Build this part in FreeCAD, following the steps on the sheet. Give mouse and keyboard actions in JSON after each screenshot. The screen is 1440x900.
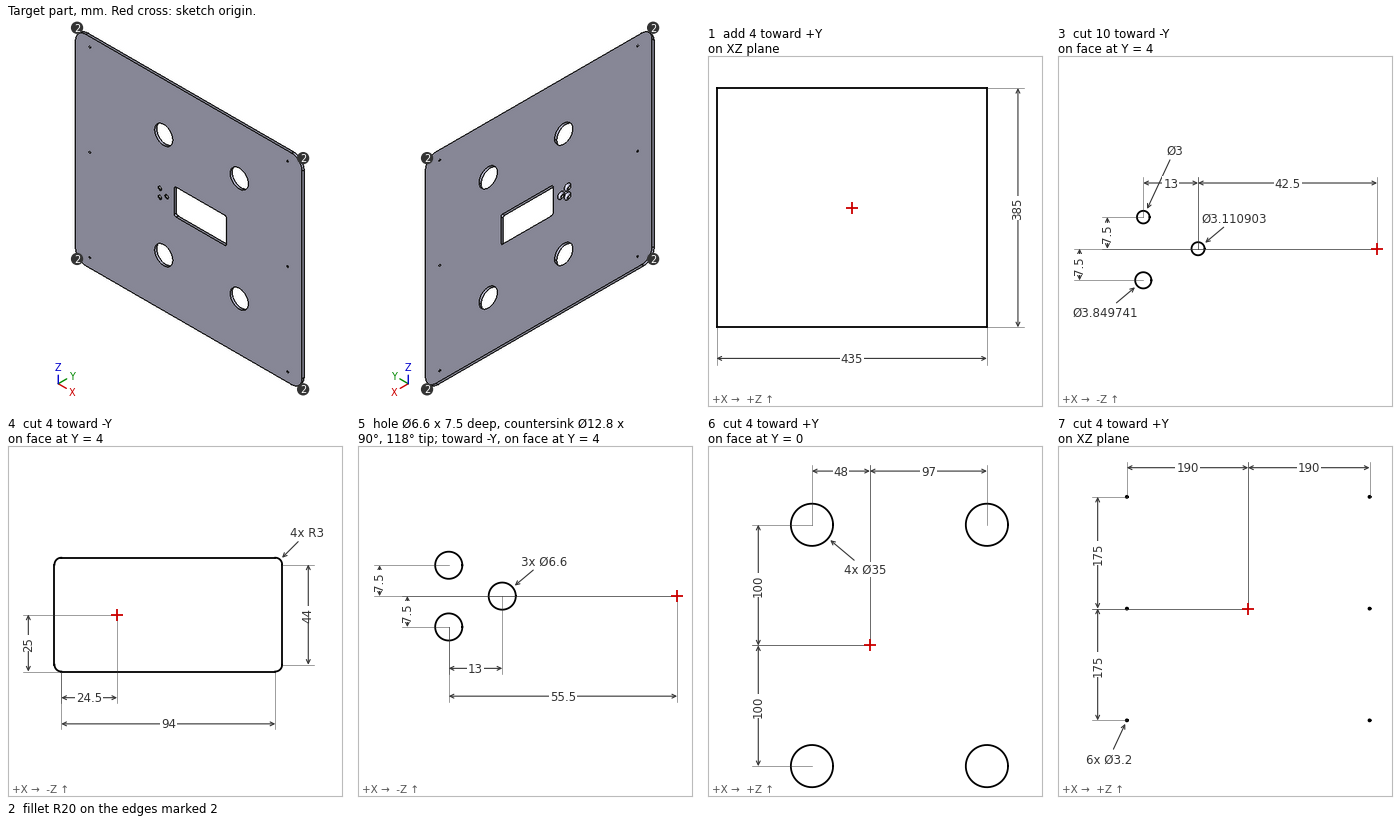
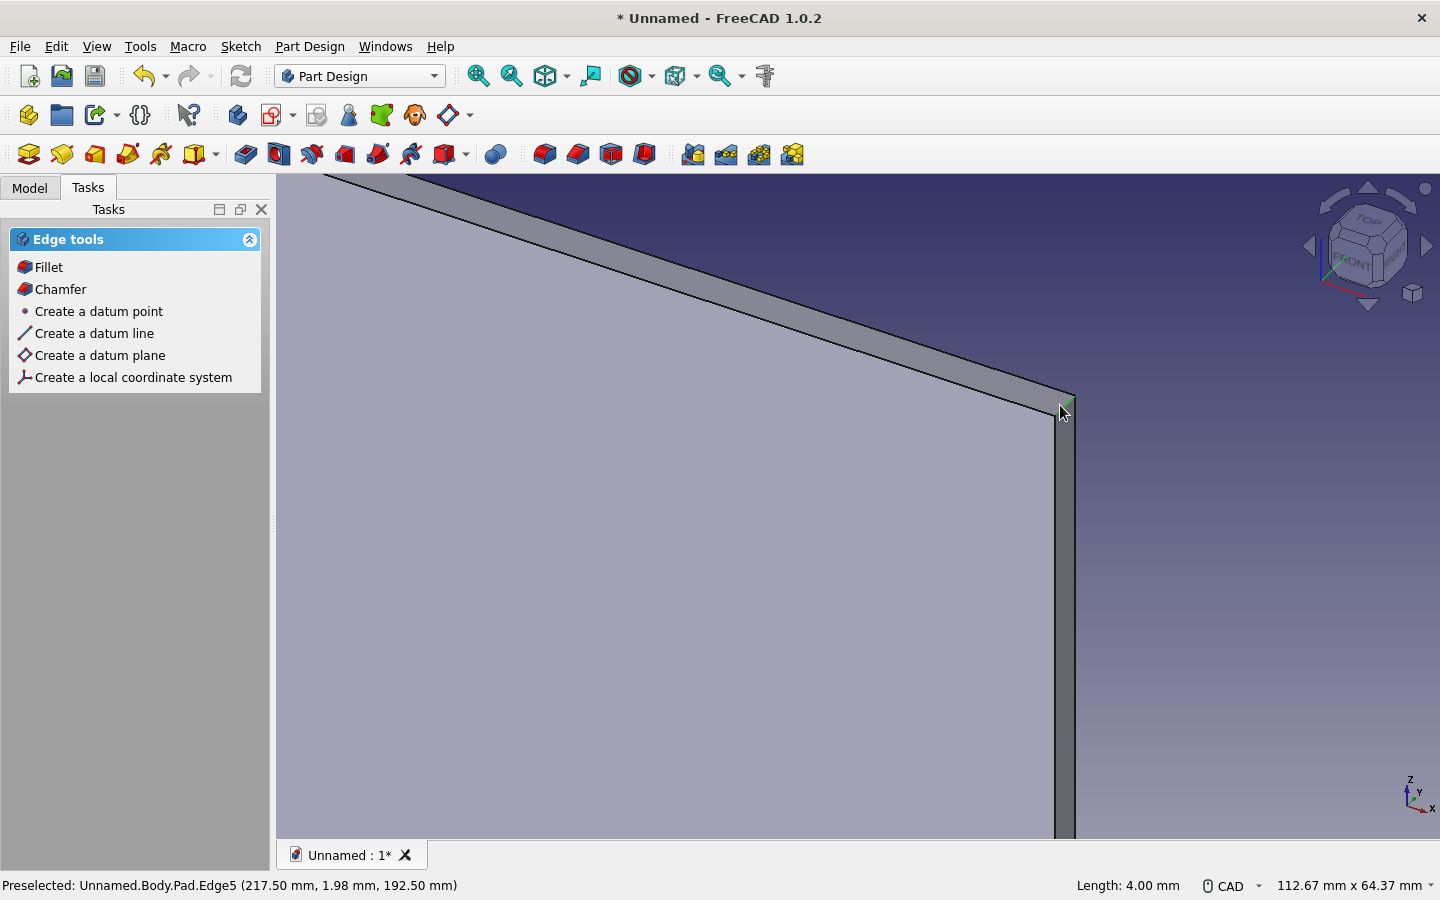
{"action": "left_click", "coordinate": [479, 76]}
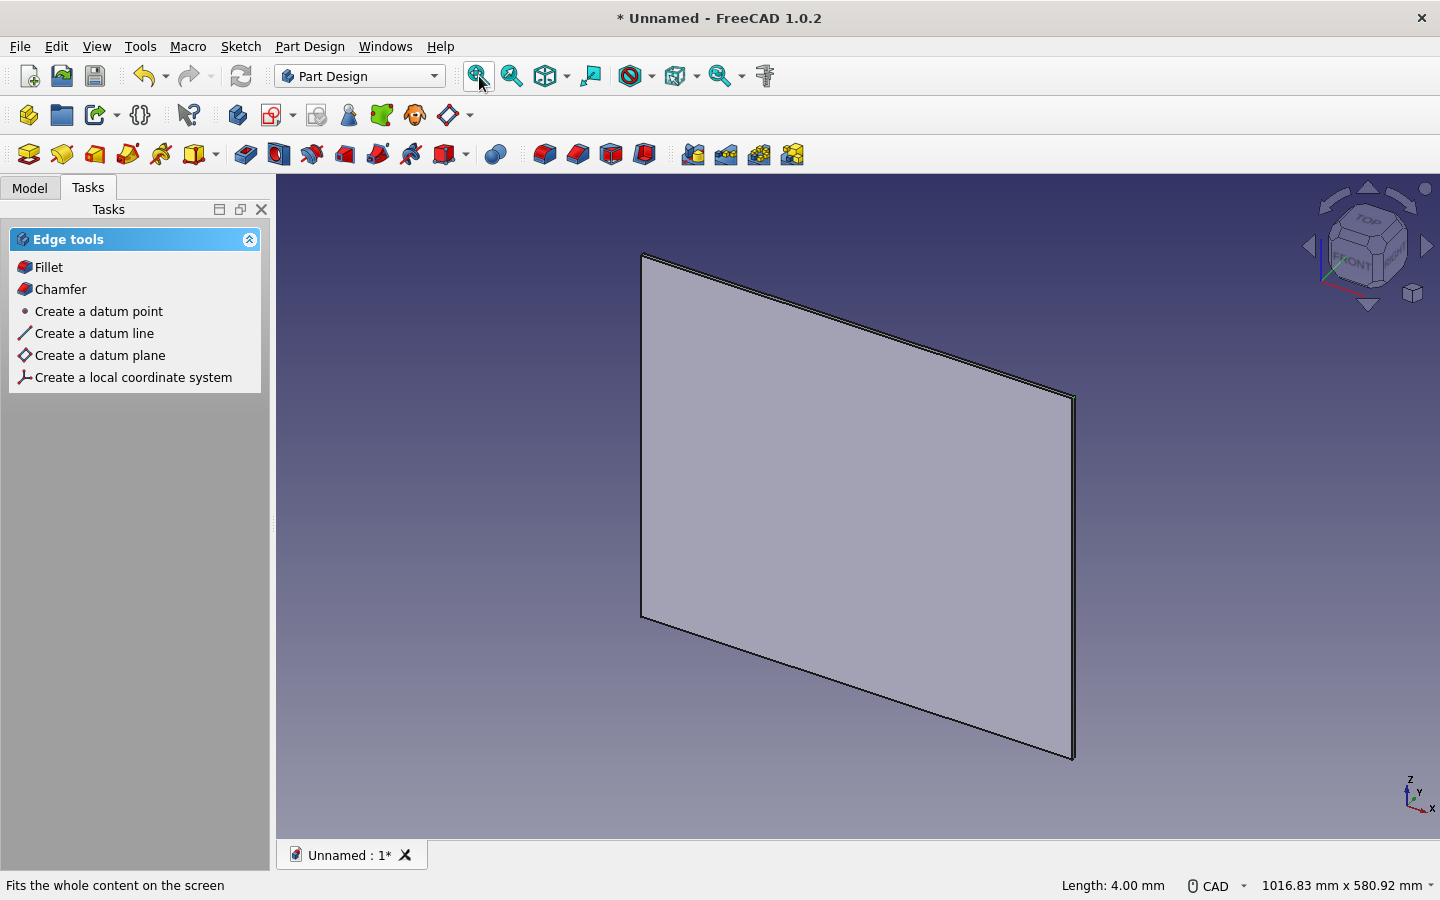
{"action": "key", "text": "0"}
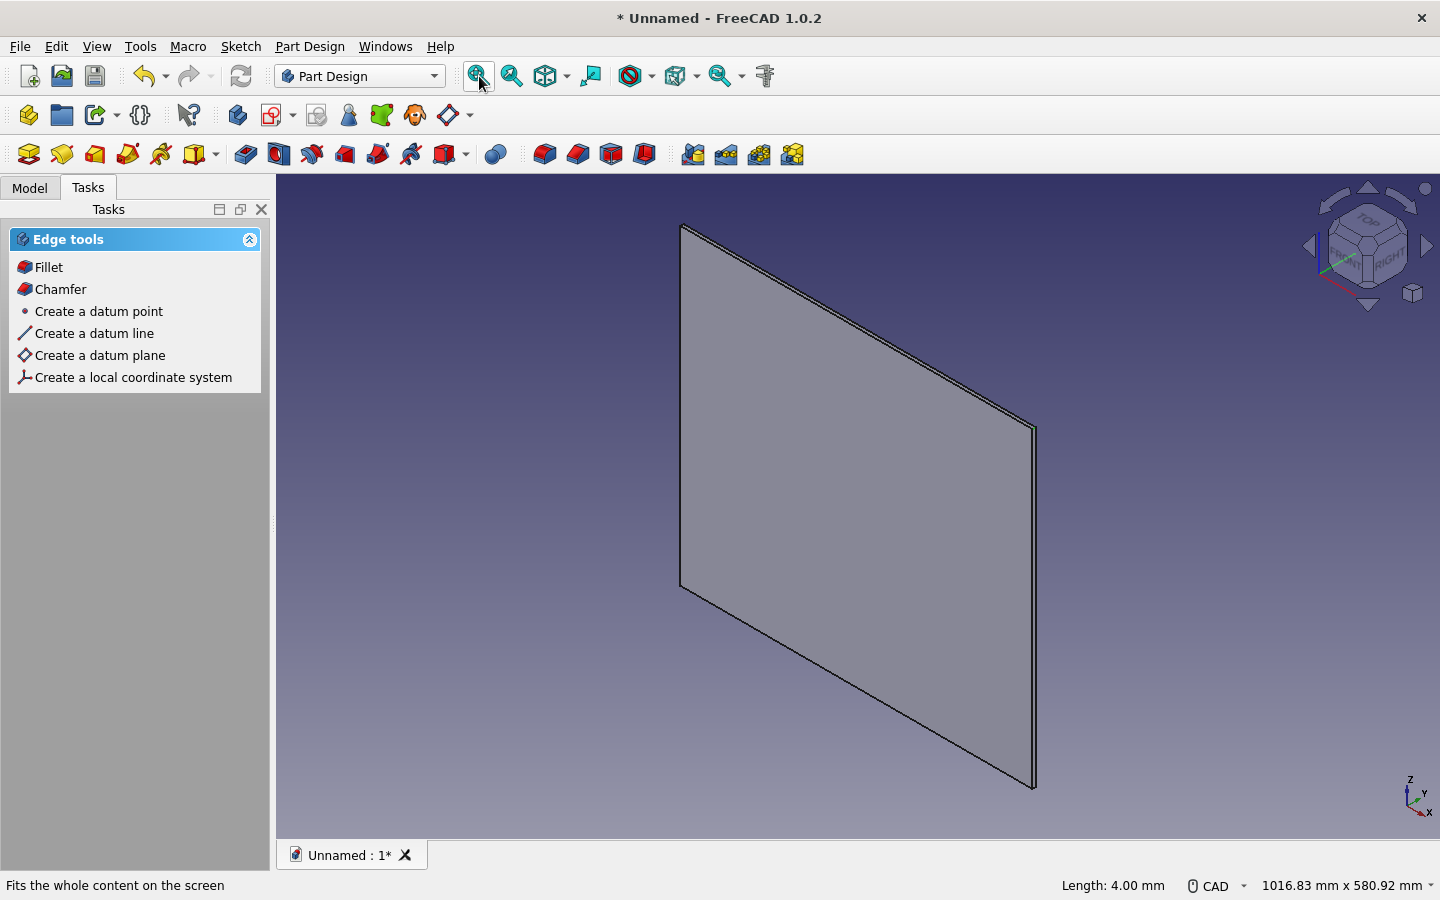
{"action": "scroll", "coordinate": [682, 224], "scroll_direction": "up", "scroll_amount": 11}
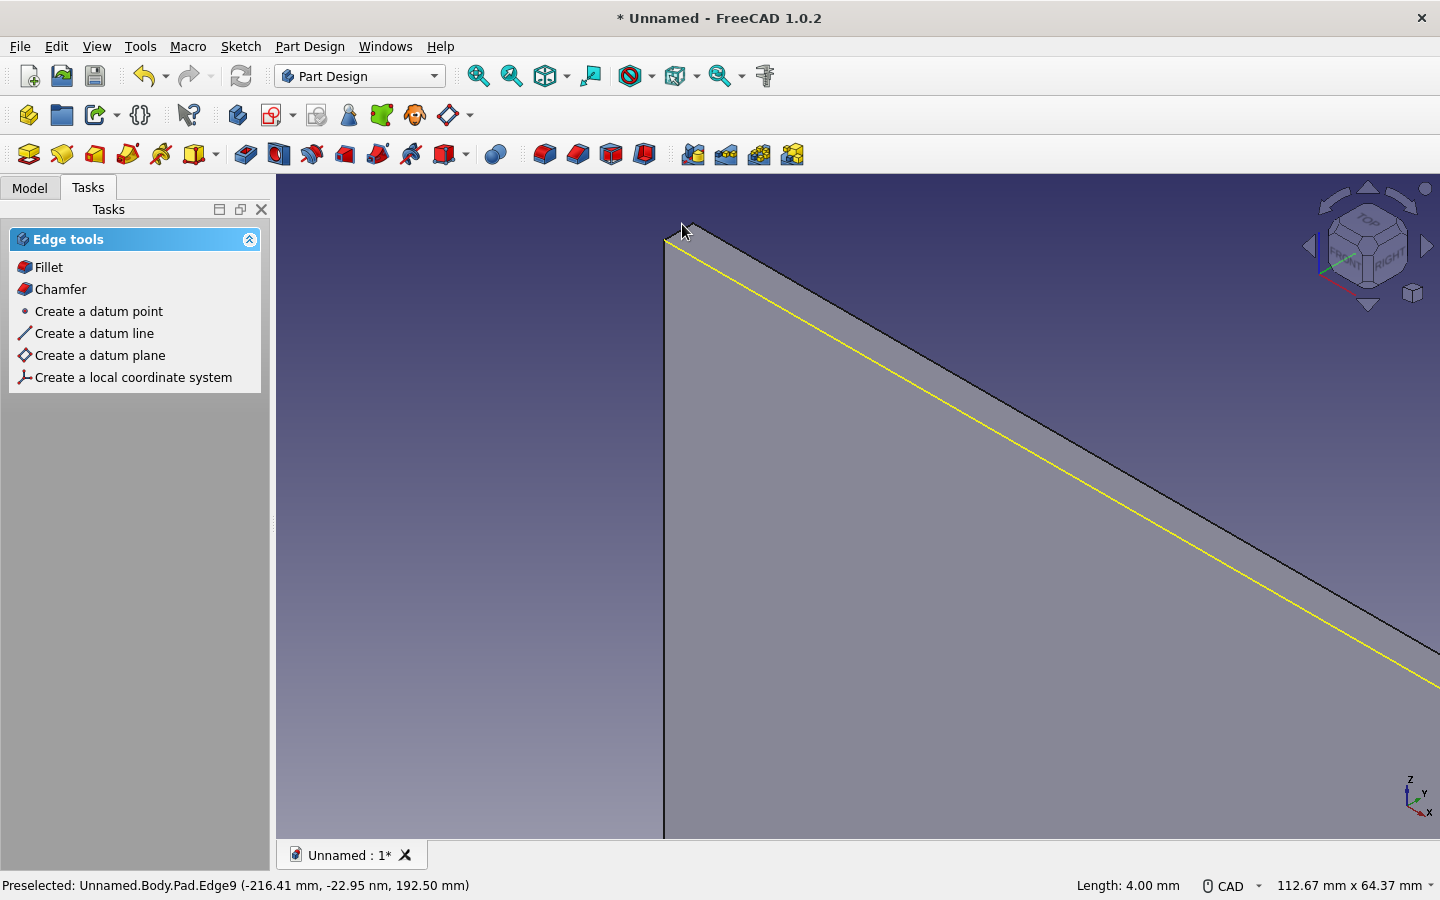
{"action": "left_click", "coordinate": [479, 76]}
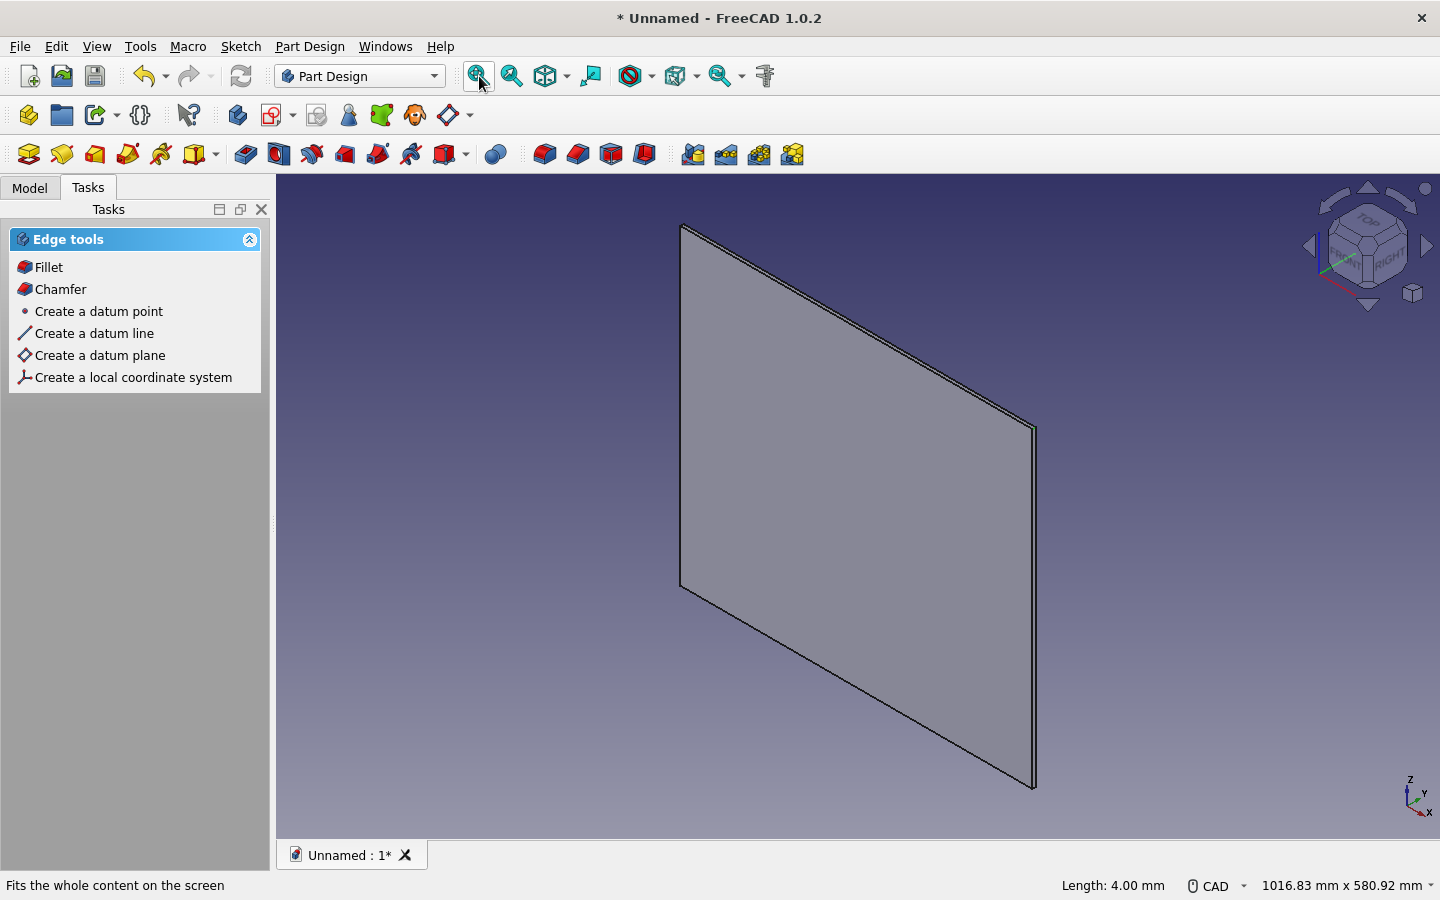
{"action": "key", "text": "2"}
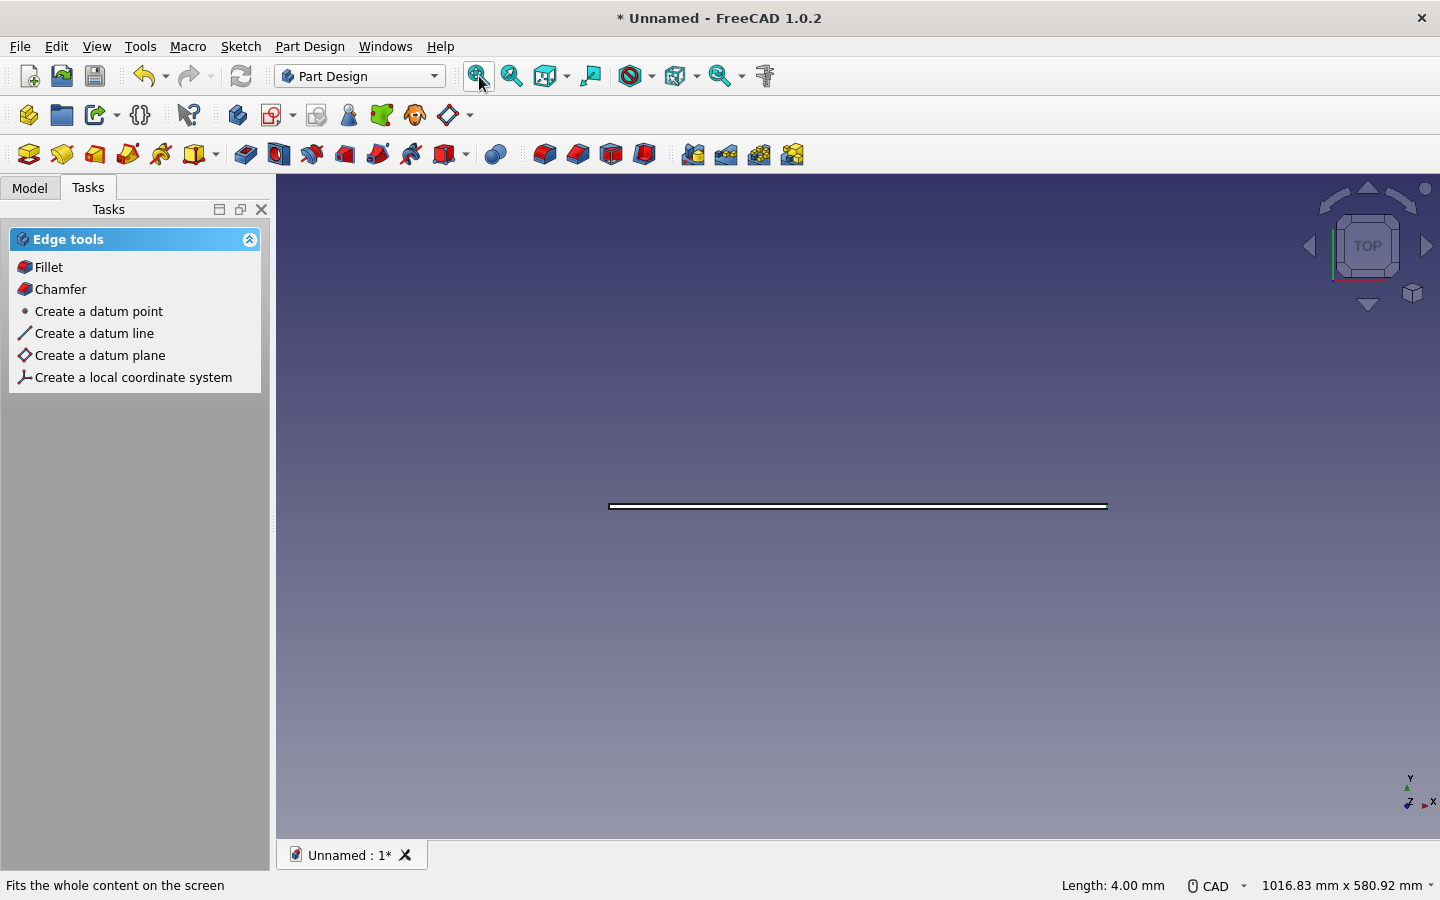
{"action": "left_click", "coordinate": [479, 76]}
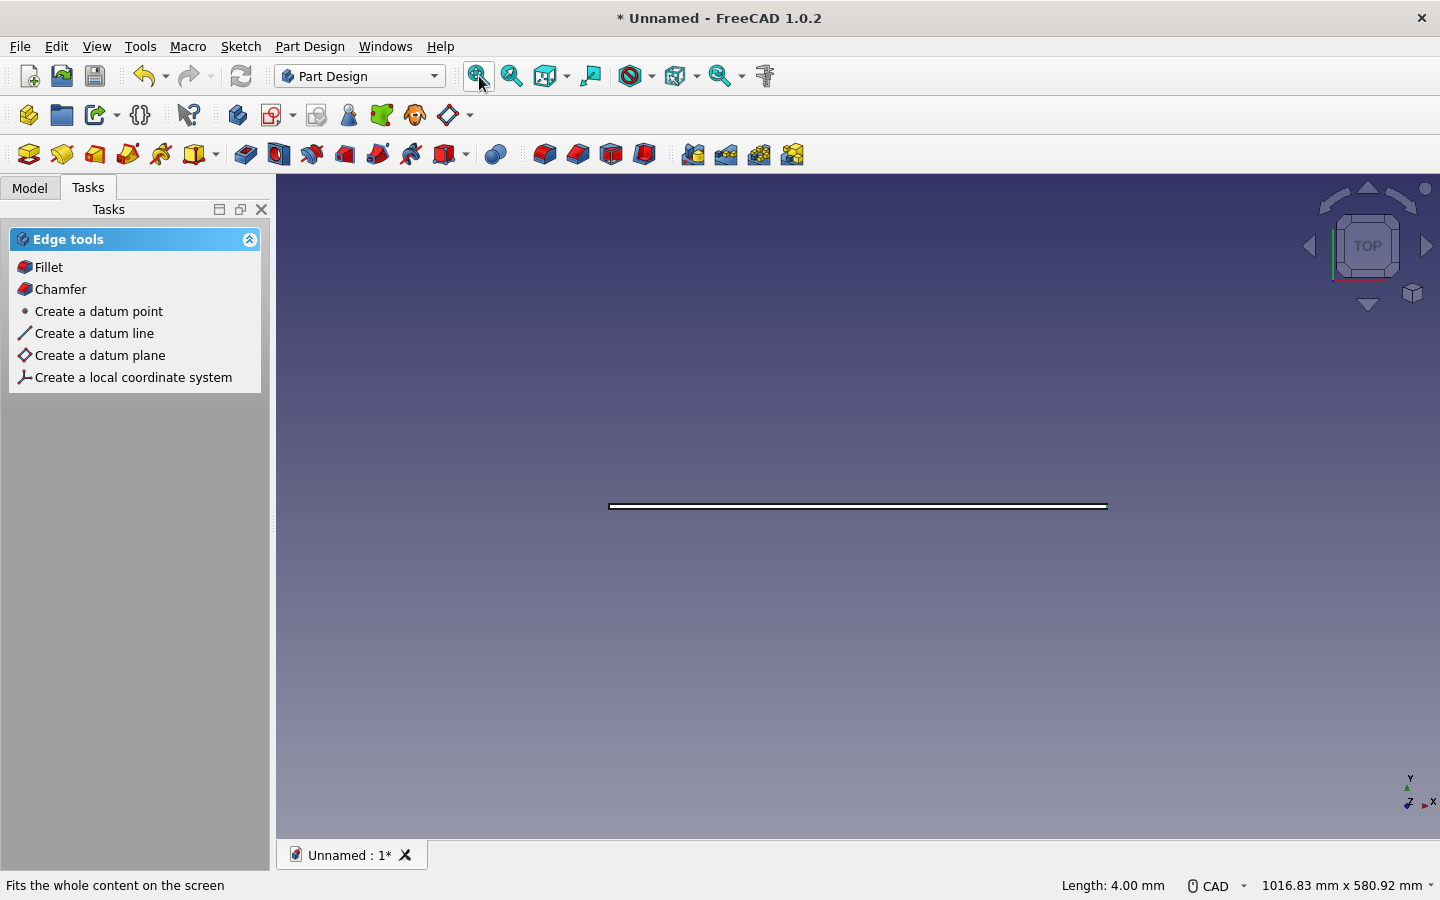
{"action": "scroll", "coordinate": [609, 505], "scroll_direction": "up", "scroll_amount": 11}